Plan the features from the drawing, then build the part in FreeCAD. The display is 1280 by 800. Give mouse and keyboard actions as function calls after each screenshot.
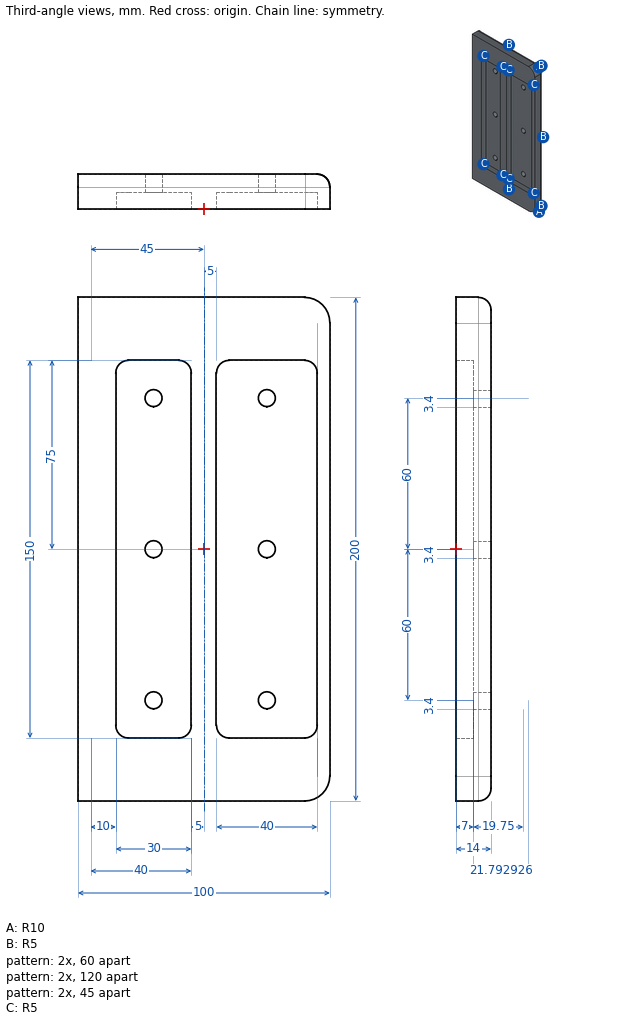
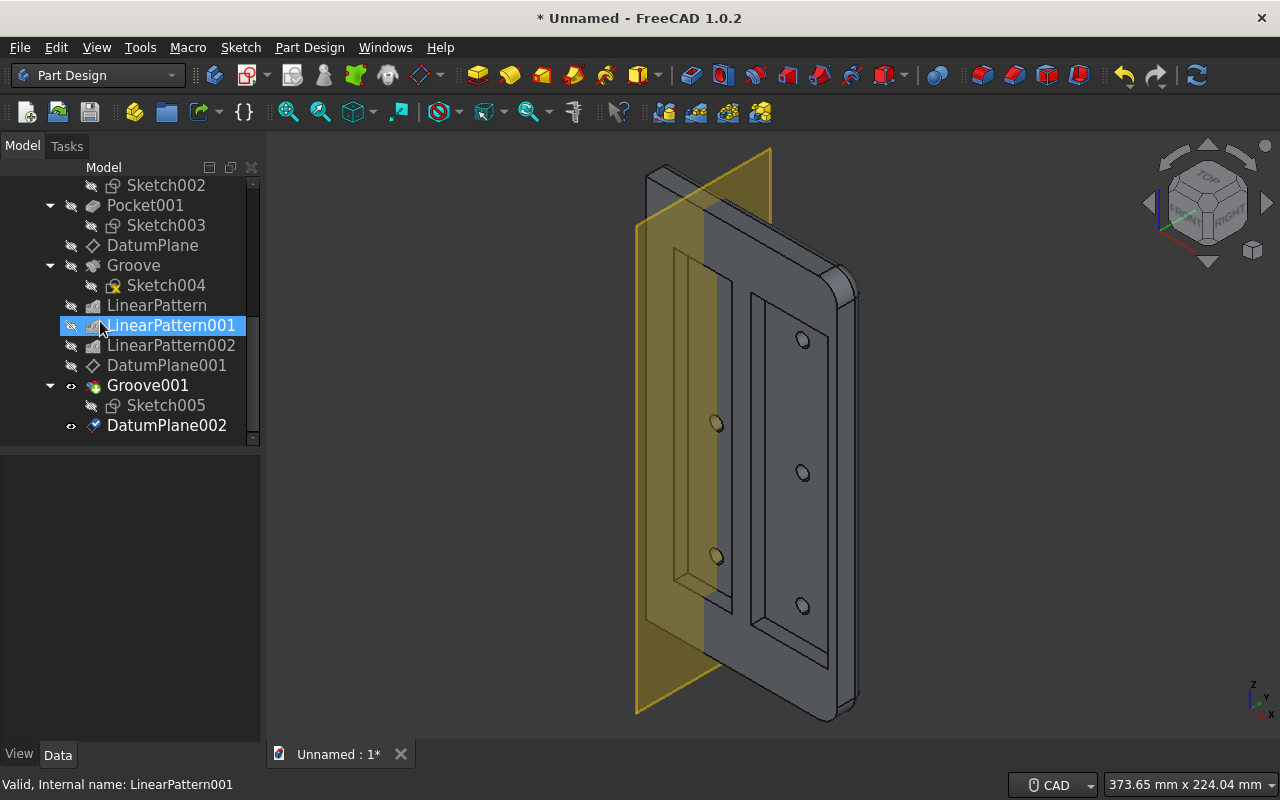
click(116, 426)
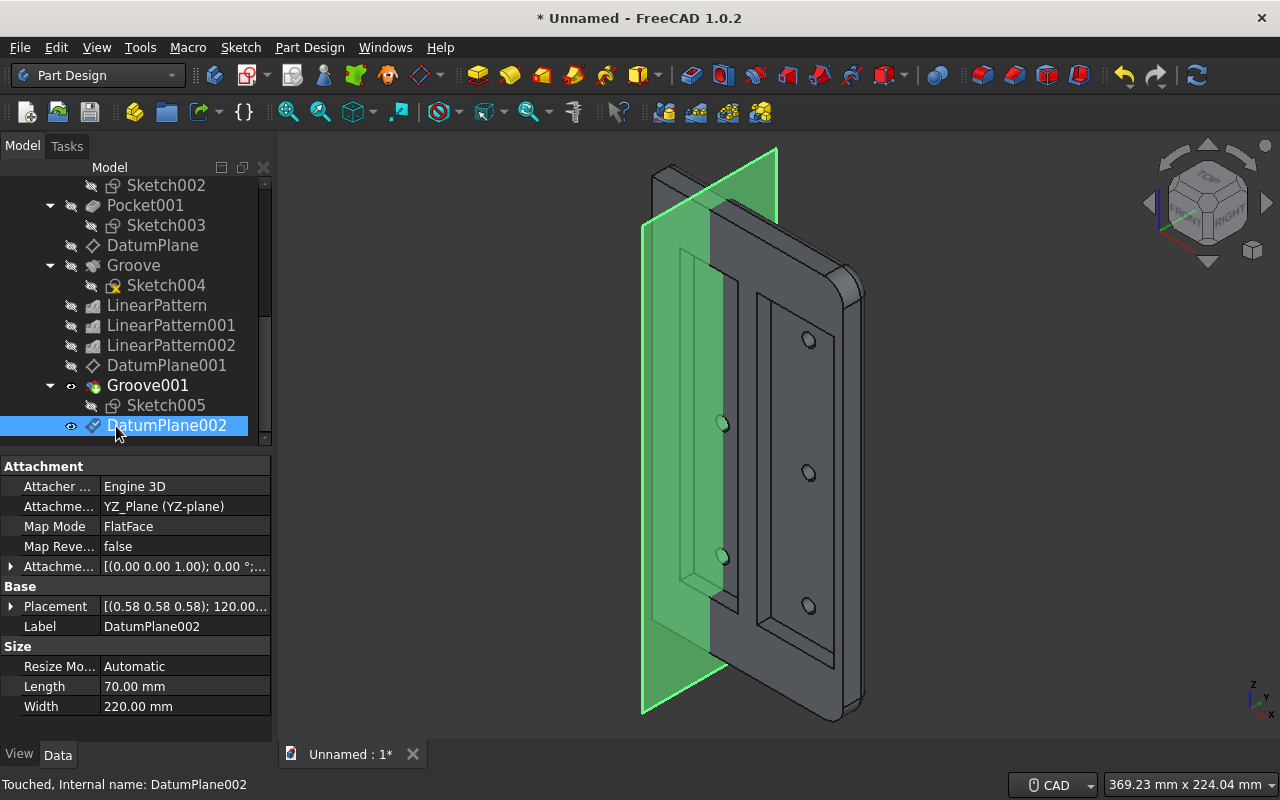
click(248, 76)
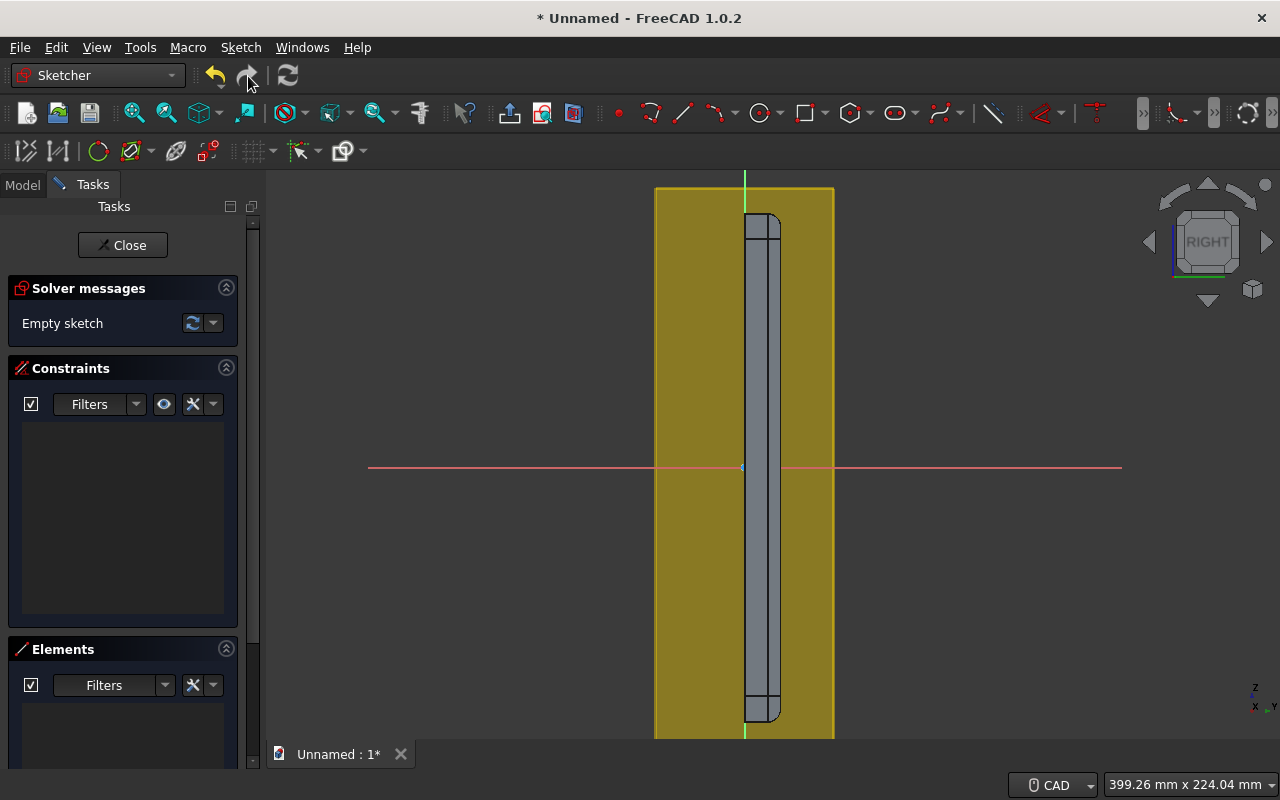
click(574, 114)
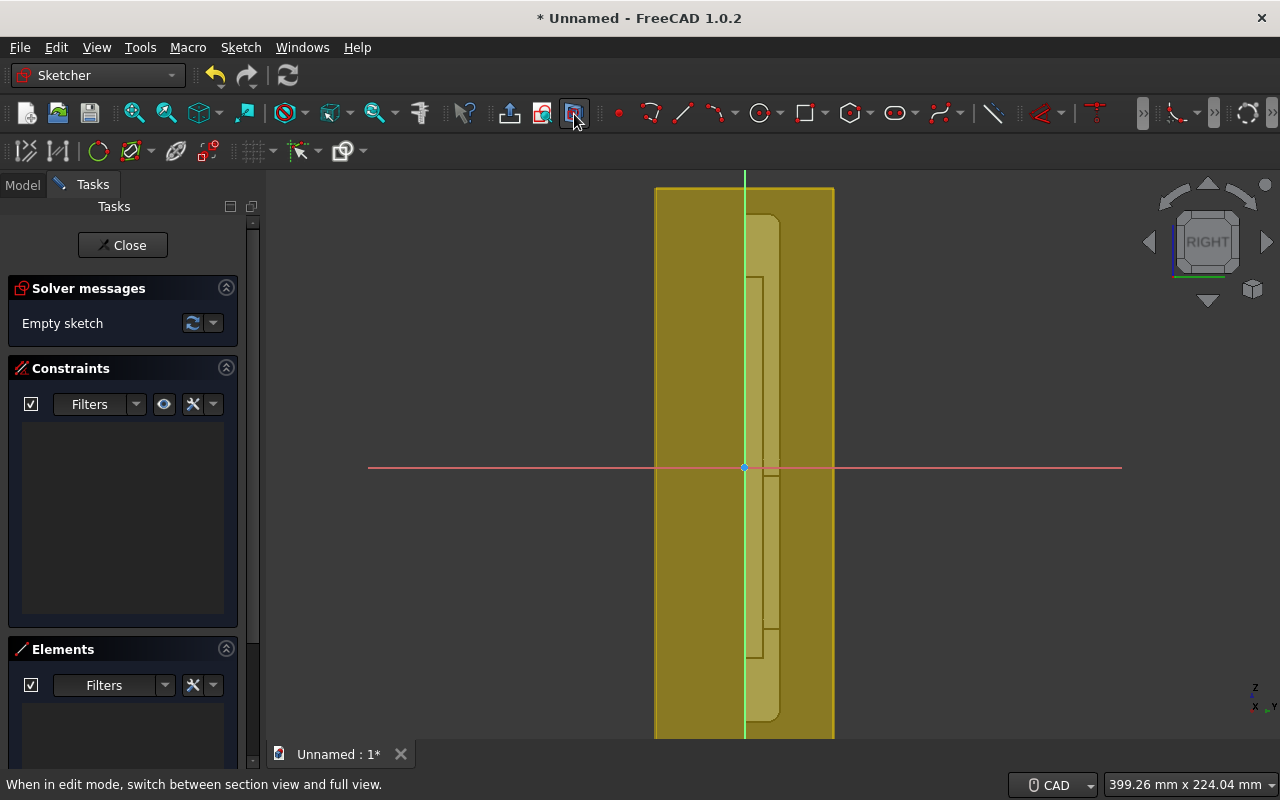
scroll(864, 340, up, 4)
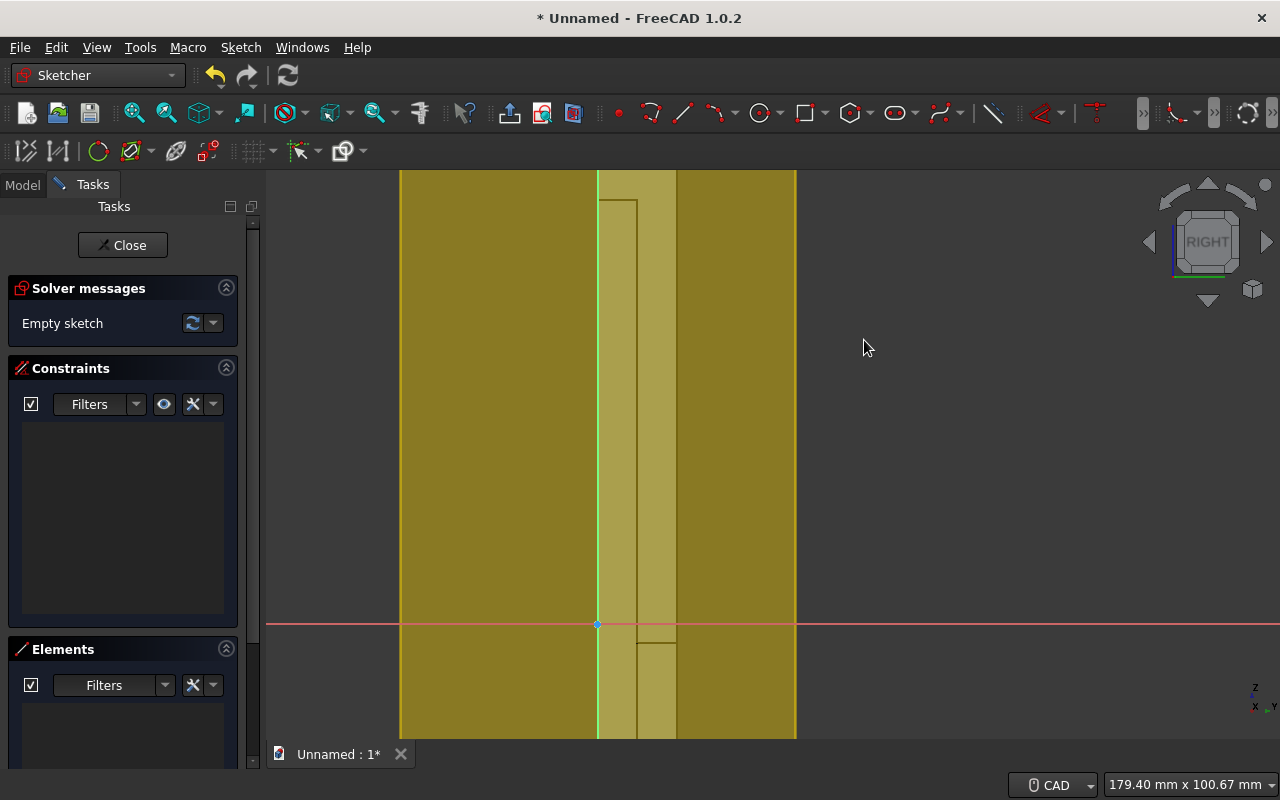
click(652, 114)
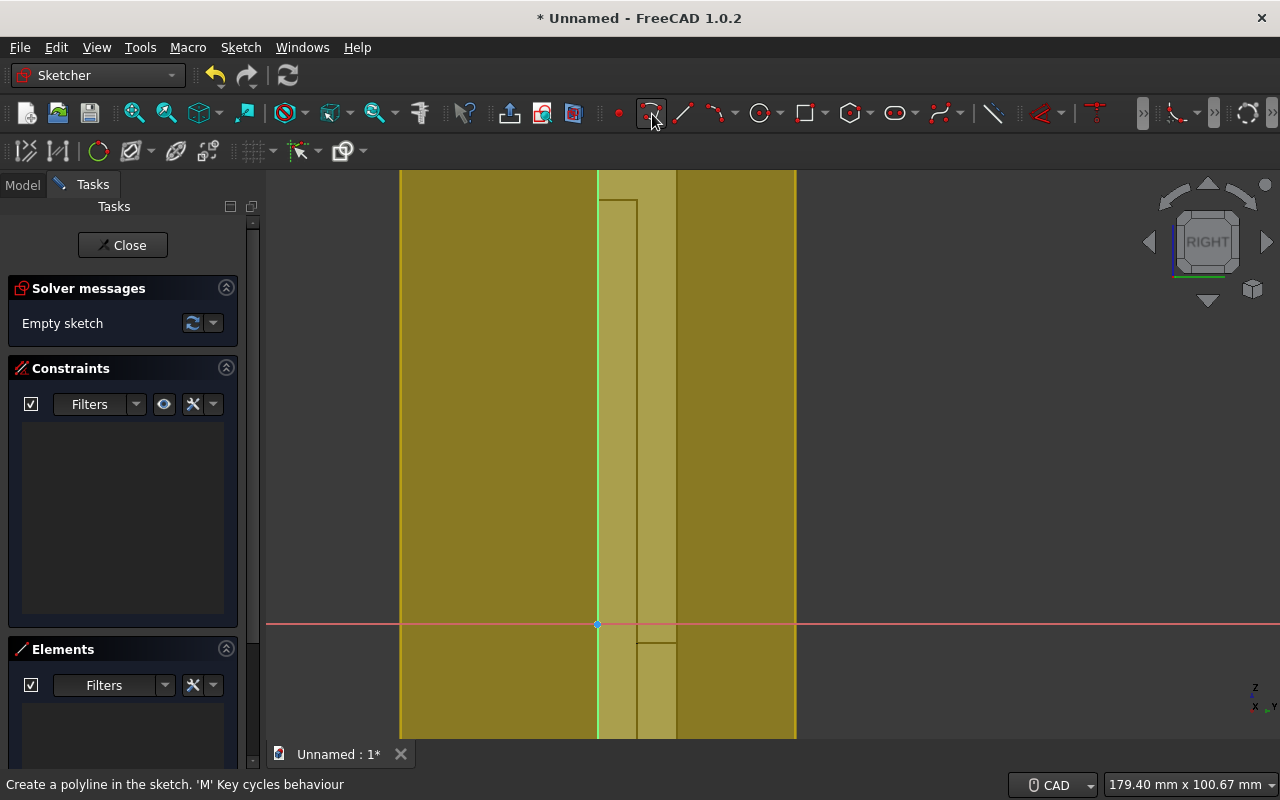
click(637, 304)
click(749, 304)
click(761, 285)
click(637, 285)
click(637, 305)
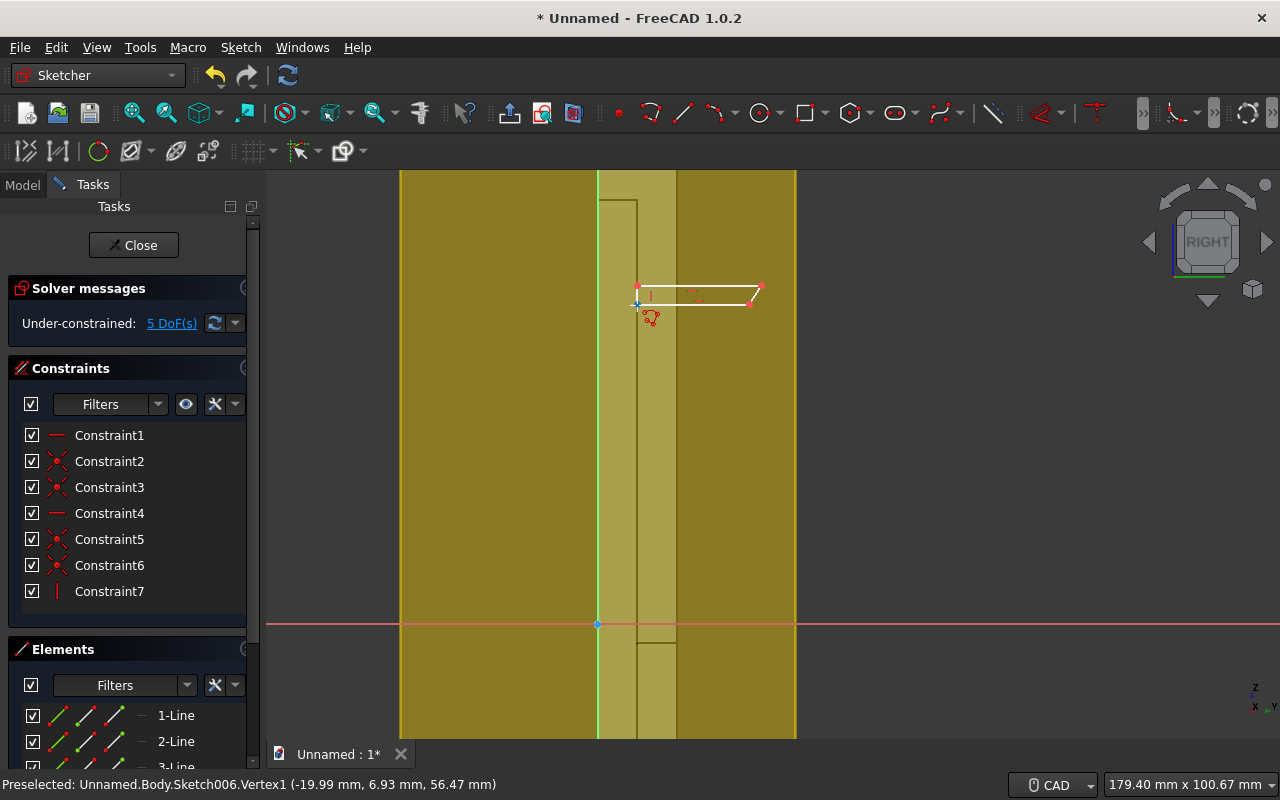
click(684, 114)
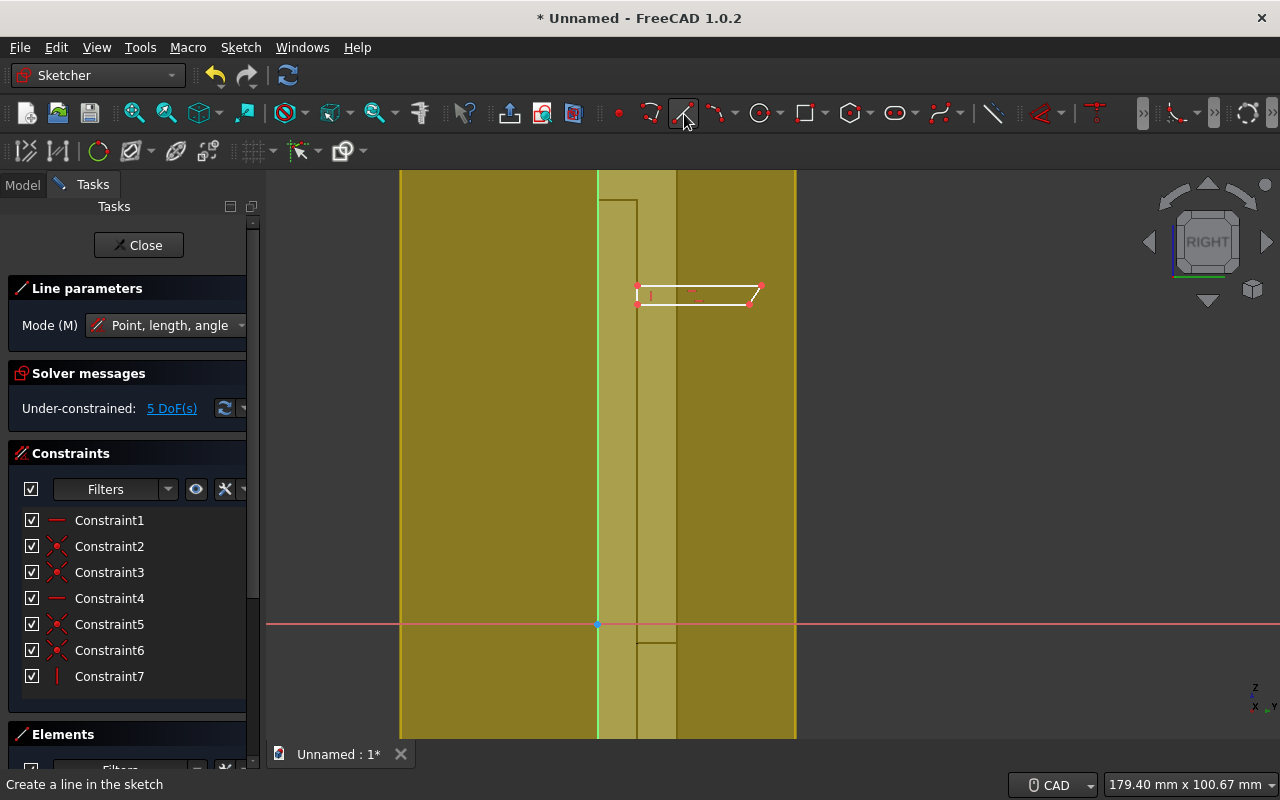
scroll(773, 285, up, 2)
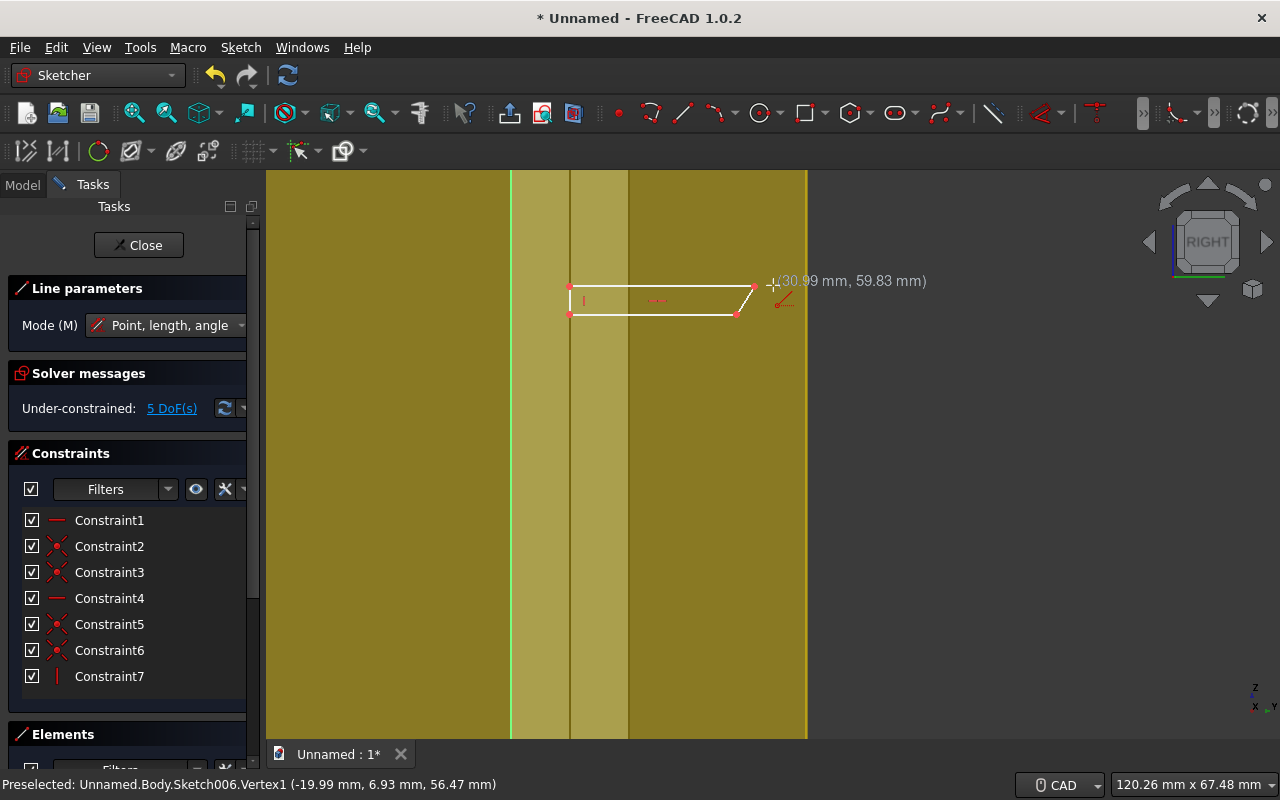
click(773, 285)
click(828, 285)
key(Escape)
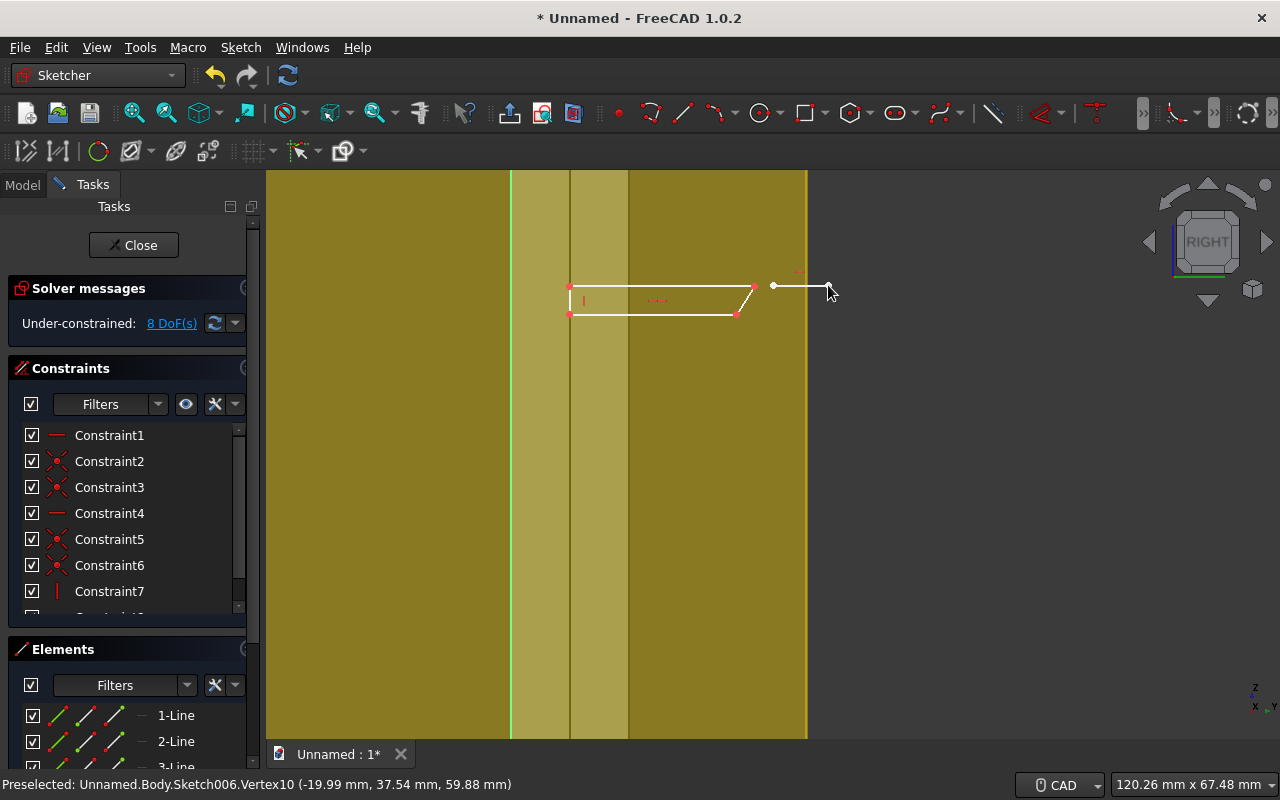
click(790, 286)